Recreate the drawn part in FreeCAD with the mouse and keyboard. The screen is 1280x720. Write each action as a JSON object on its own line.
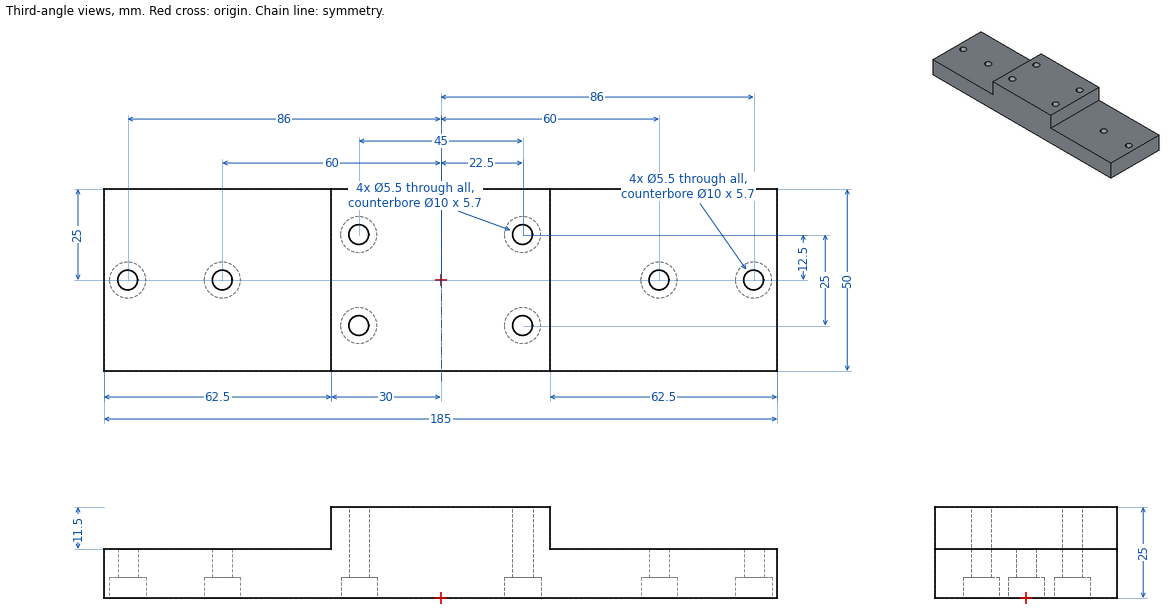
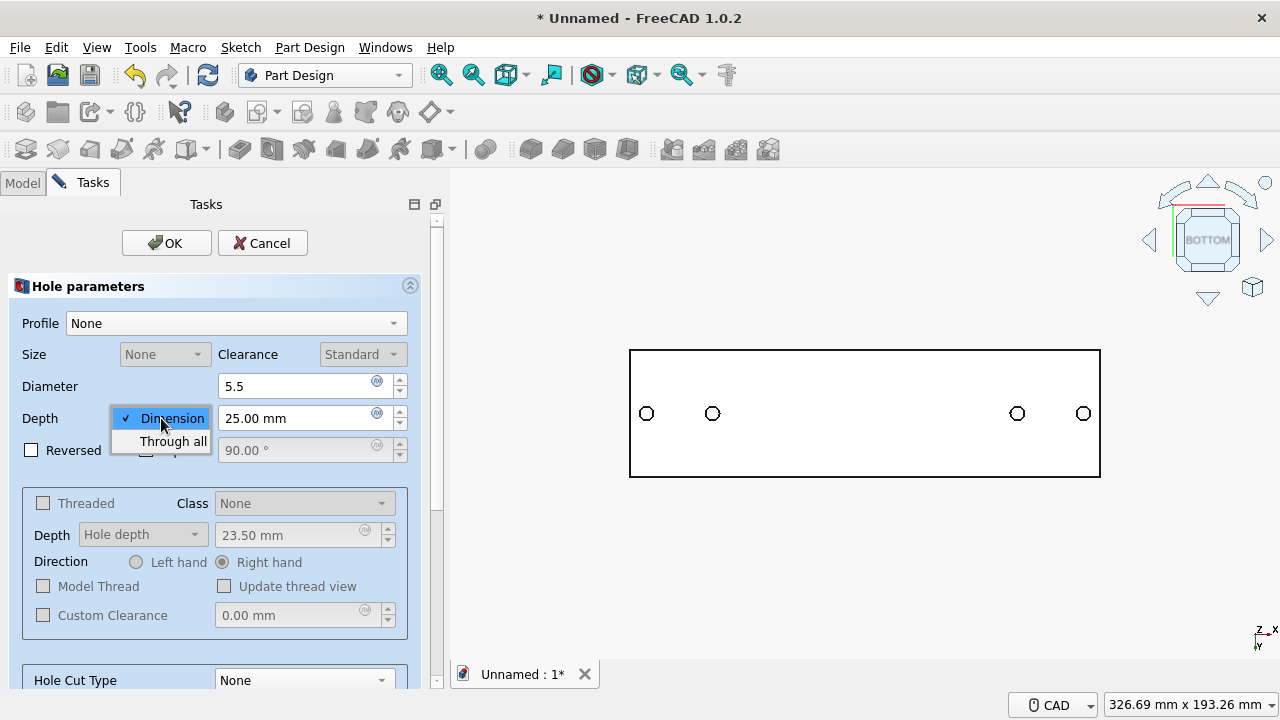
{"action": "left_click", "coordinate": [160, 442]}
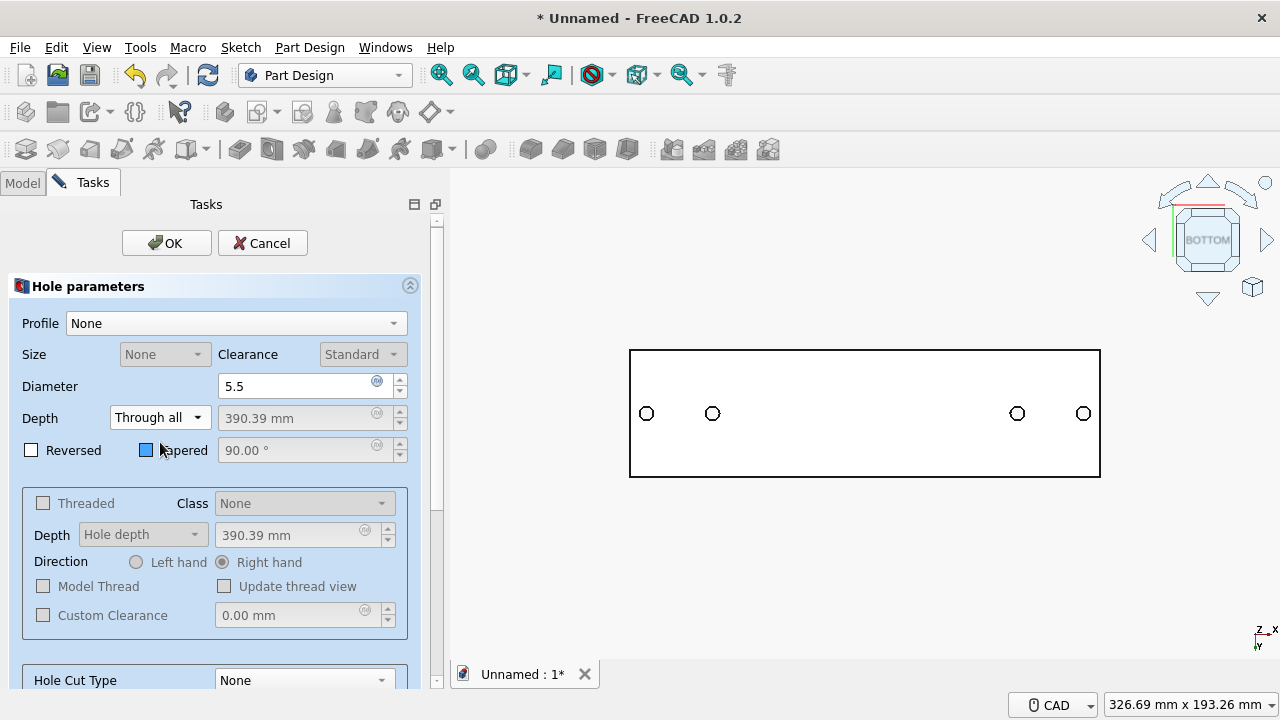
{"action": "scroll", "coordinate": [437, 451], "scroll_direction": "down", "scroll_amount": 2}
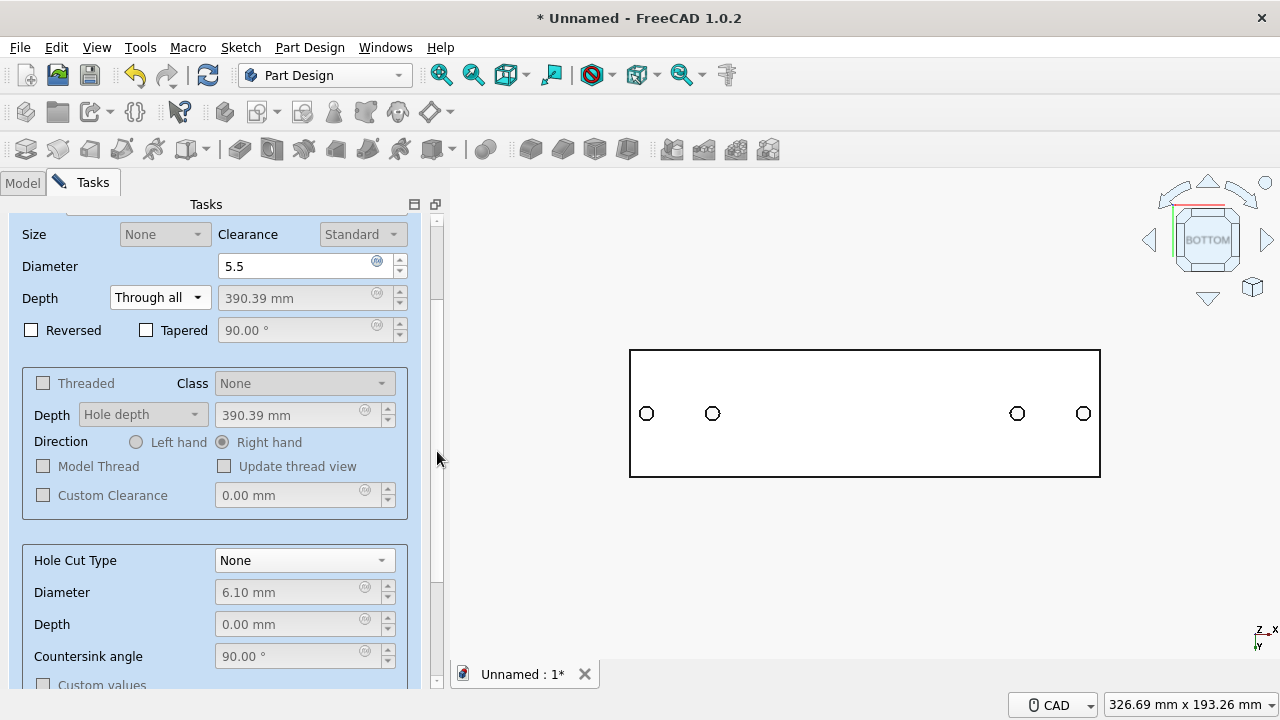
{"action": "left_click", "coordinate": [306, 560]}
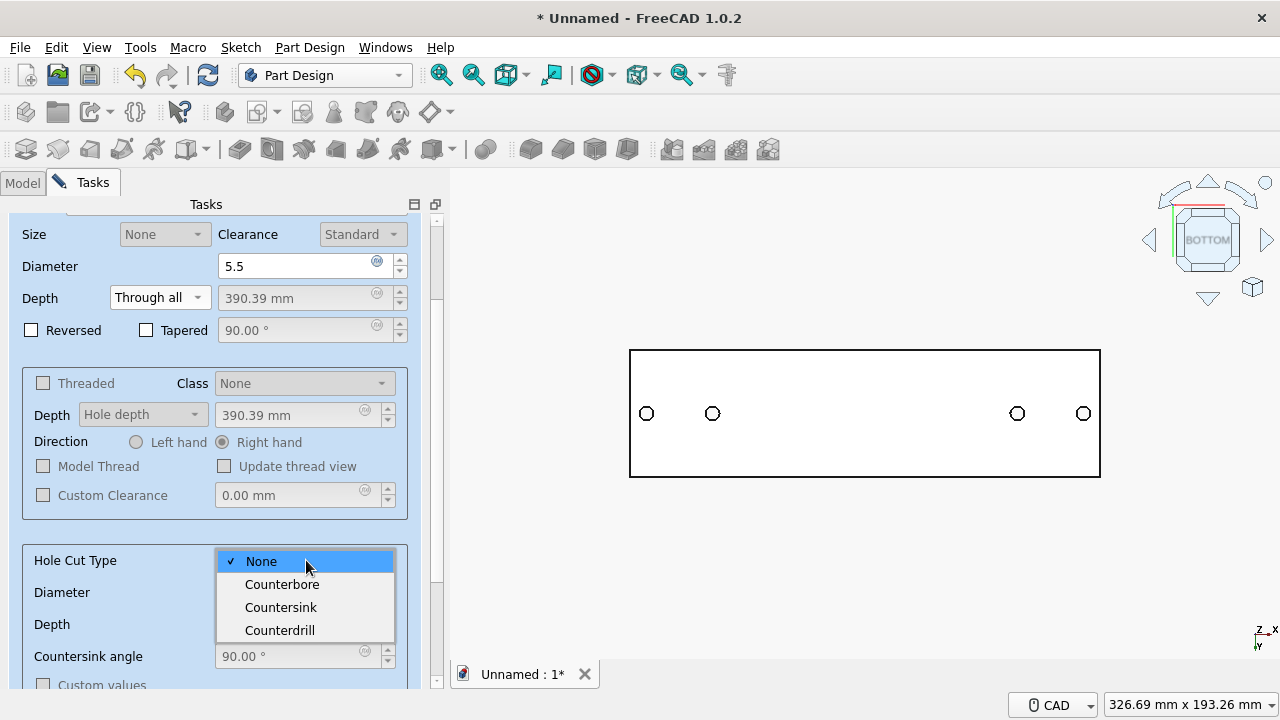
{"action": "left_click", "coordinate": [304, 584]}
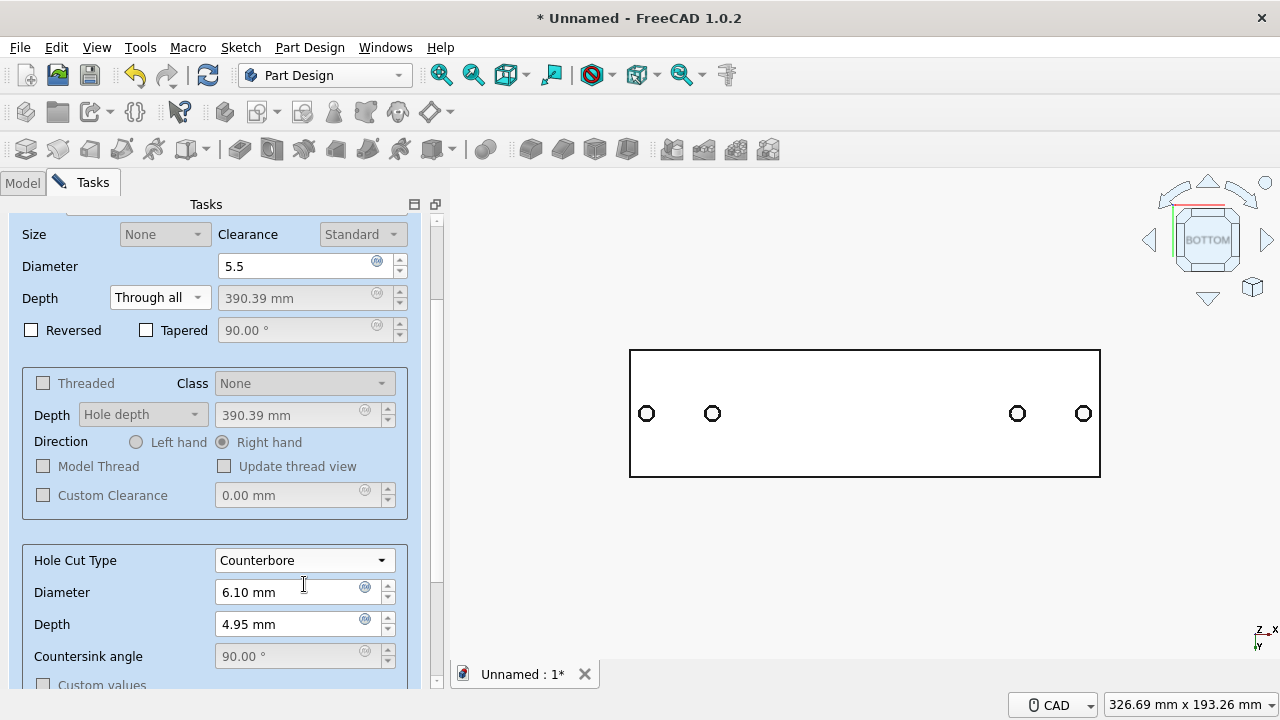
{"action": "triple_click", "coordinate": [298, 592]}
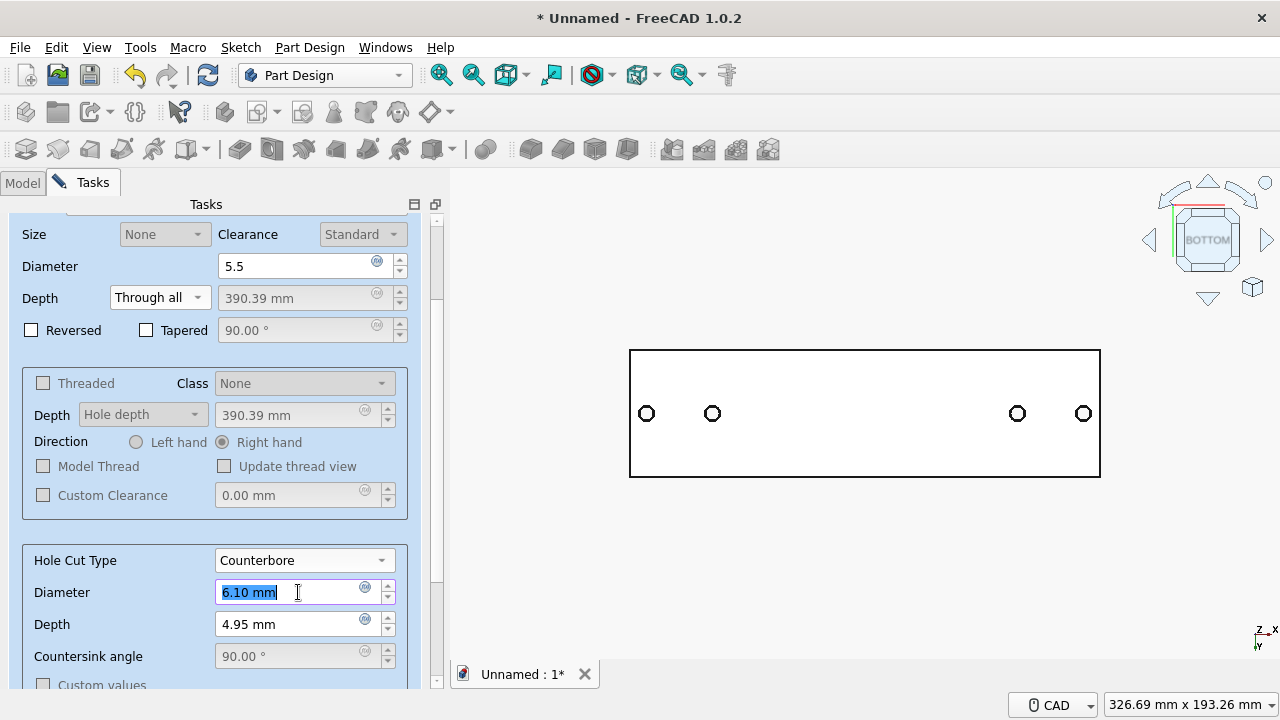
{"action": "type", "text": "10"}
{"action": "key", "text": "Tab"}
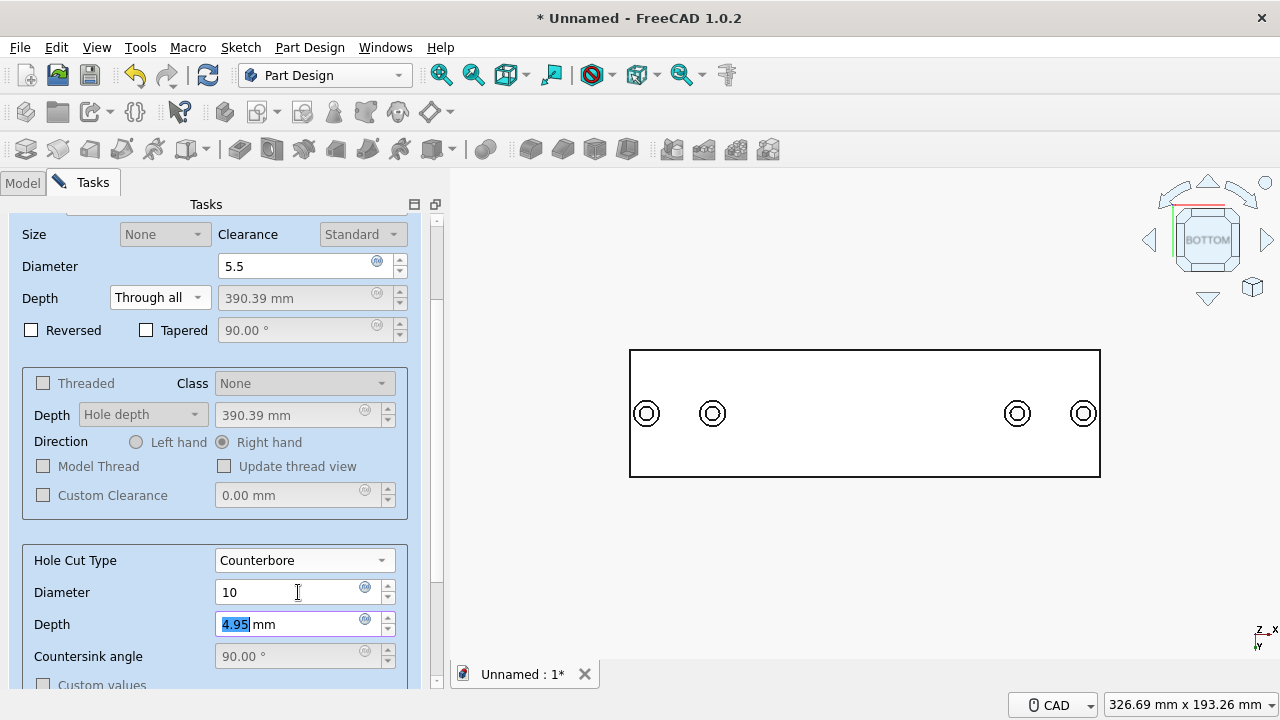
{"action": "type", "text": "5.7"}
{"action": "key", "text": "Tab"}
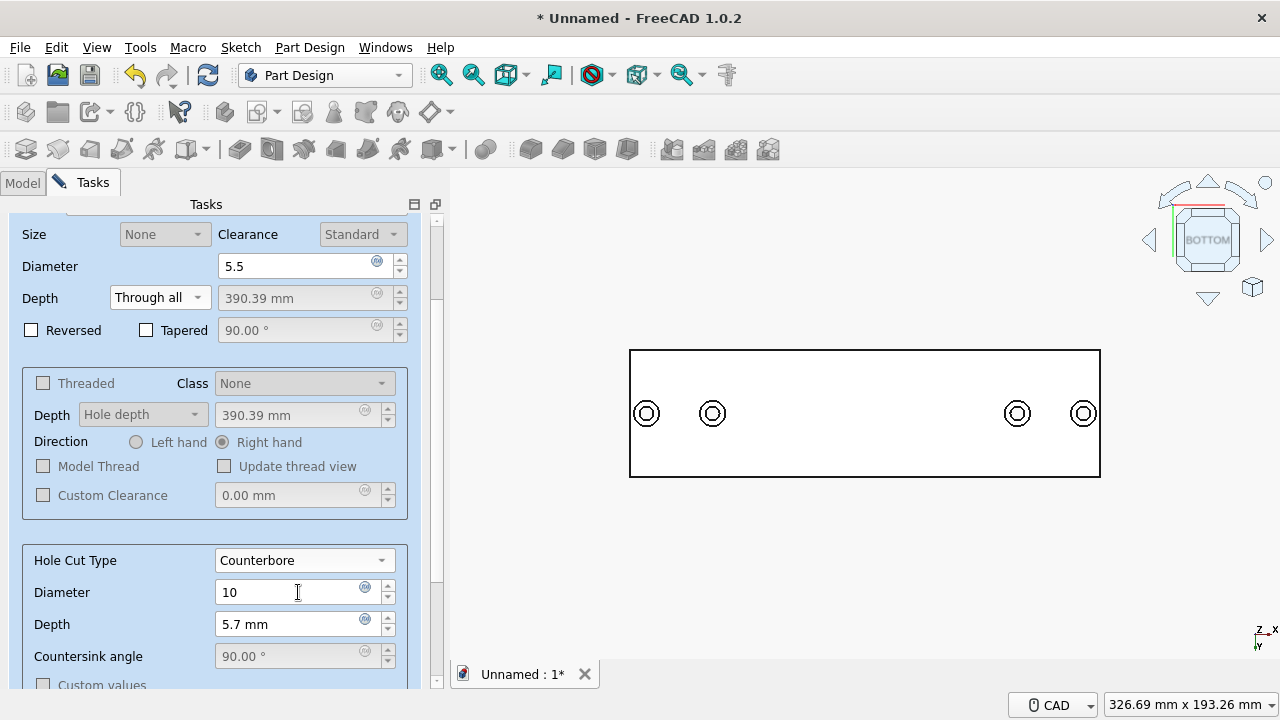
{"action": "scroll", "coordinate": [437, 451], "scroll_direction": "up", "scroll_amount": 3}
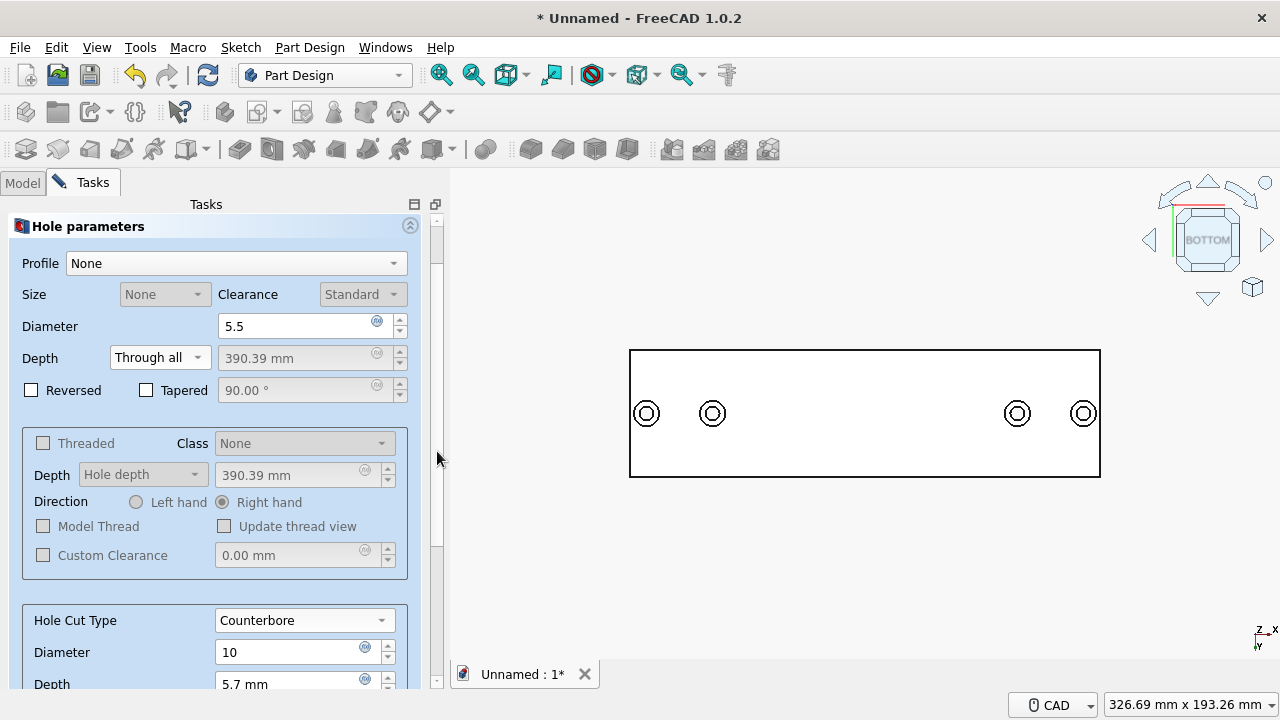
{"action": "left_click", "coordinate": [167, 243]}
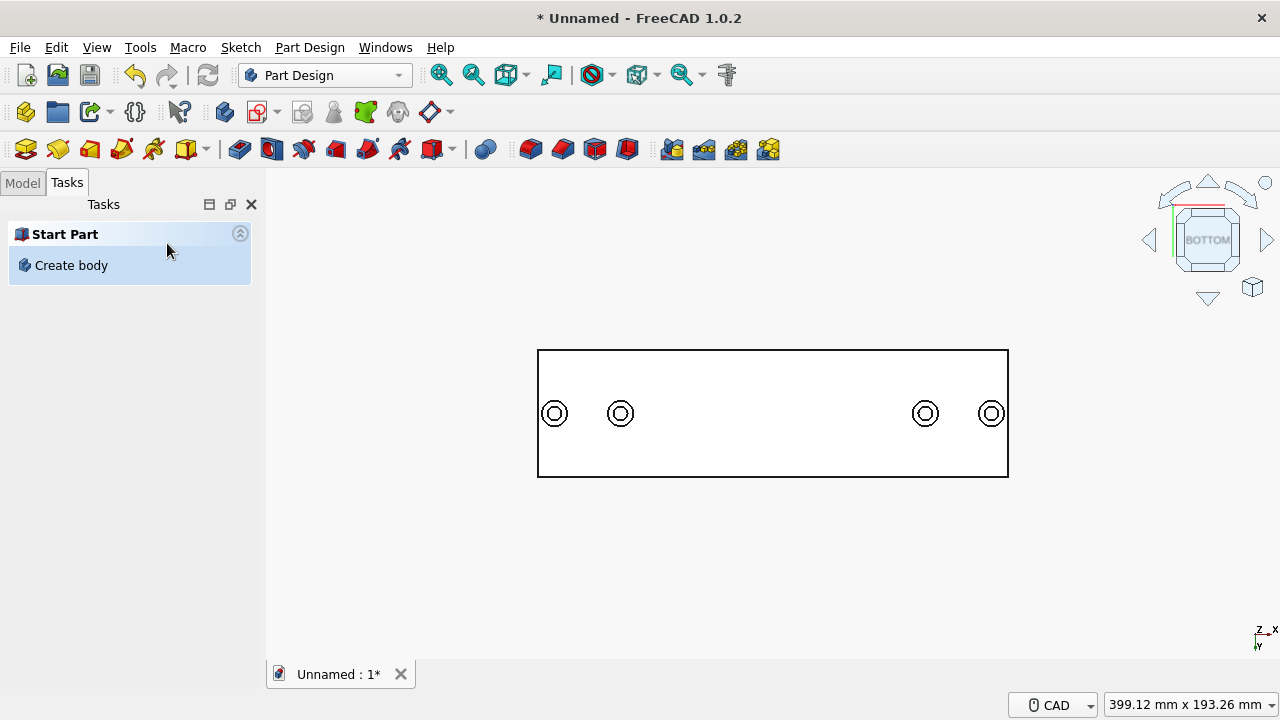
{"action": "left_click", "coordinate": [258, 112]}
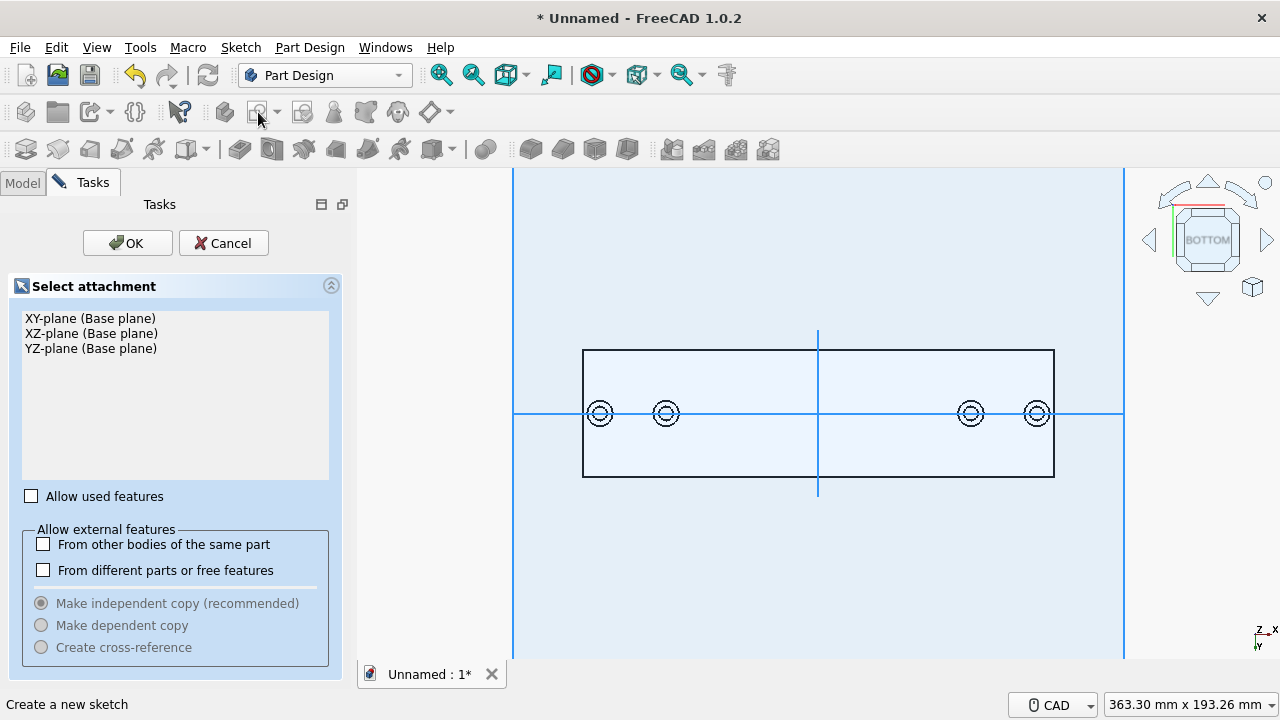
{"action": "left_click", "coordinate": [82, 318]}